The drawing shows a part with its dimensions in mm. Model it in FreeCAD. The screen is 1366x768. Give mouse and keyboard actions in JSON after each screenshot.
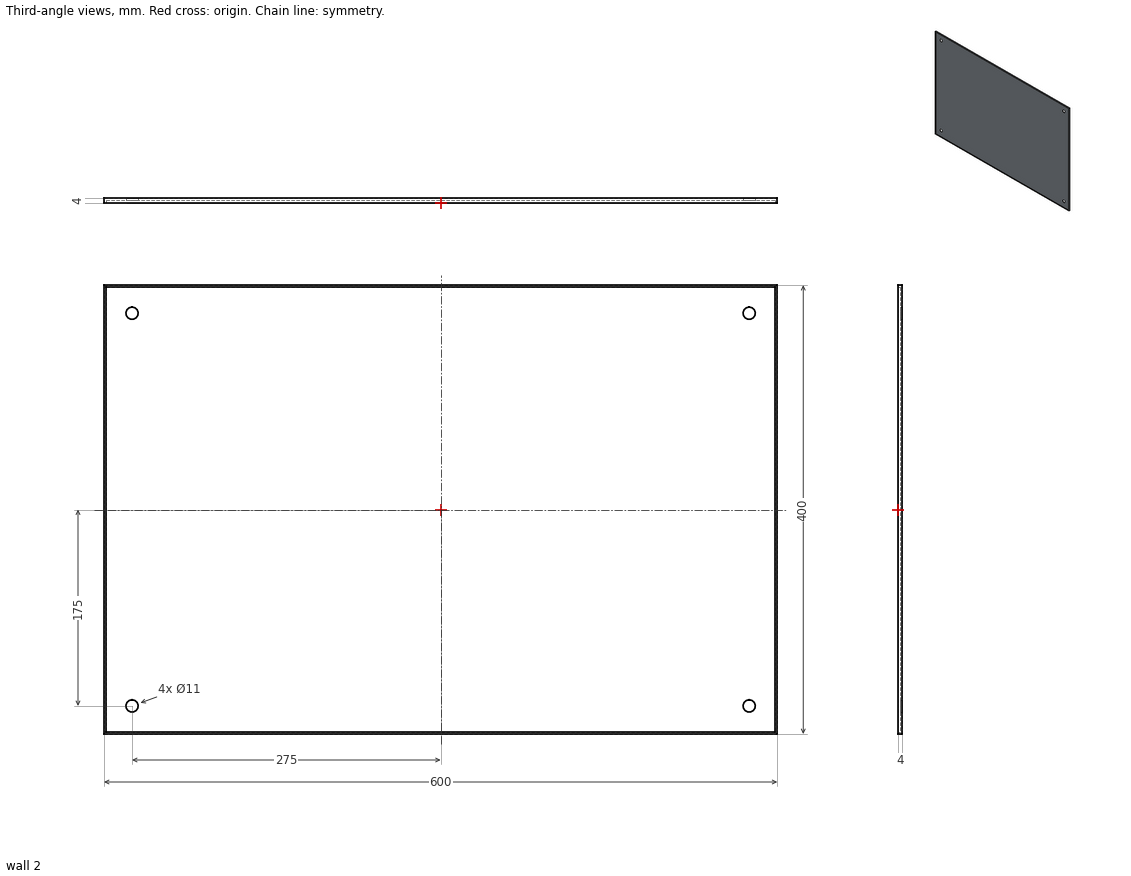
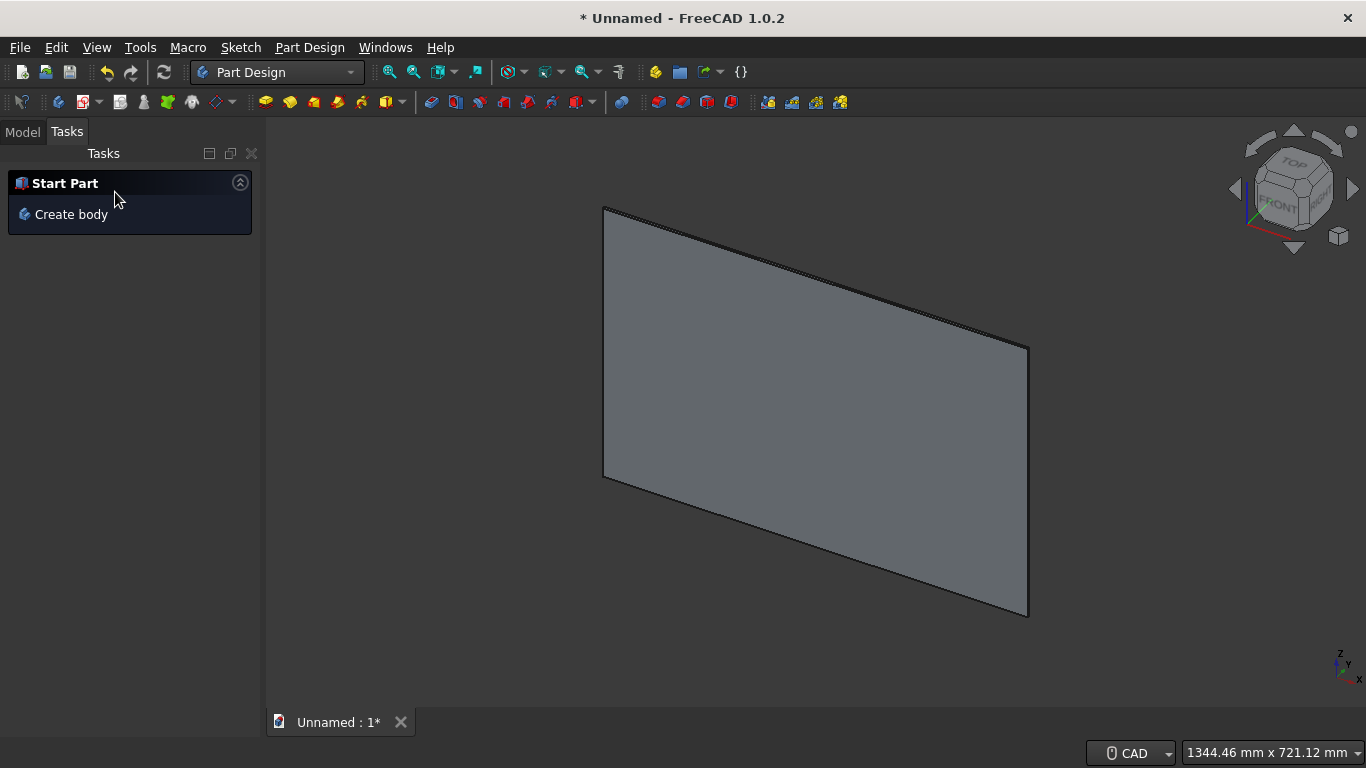
{"action": "left_click", "coordinate": [876, 432]}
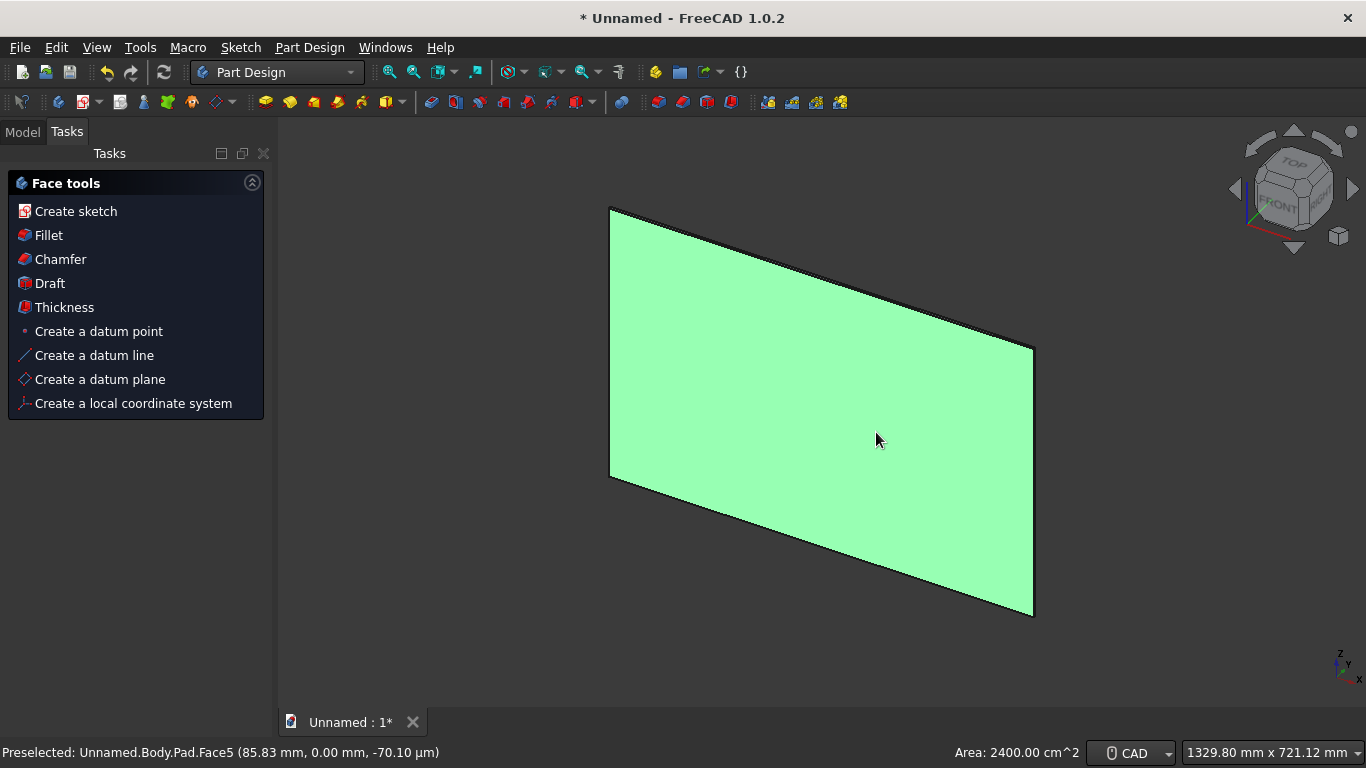
{"action": "left_click", "coordinate": [732, 102]}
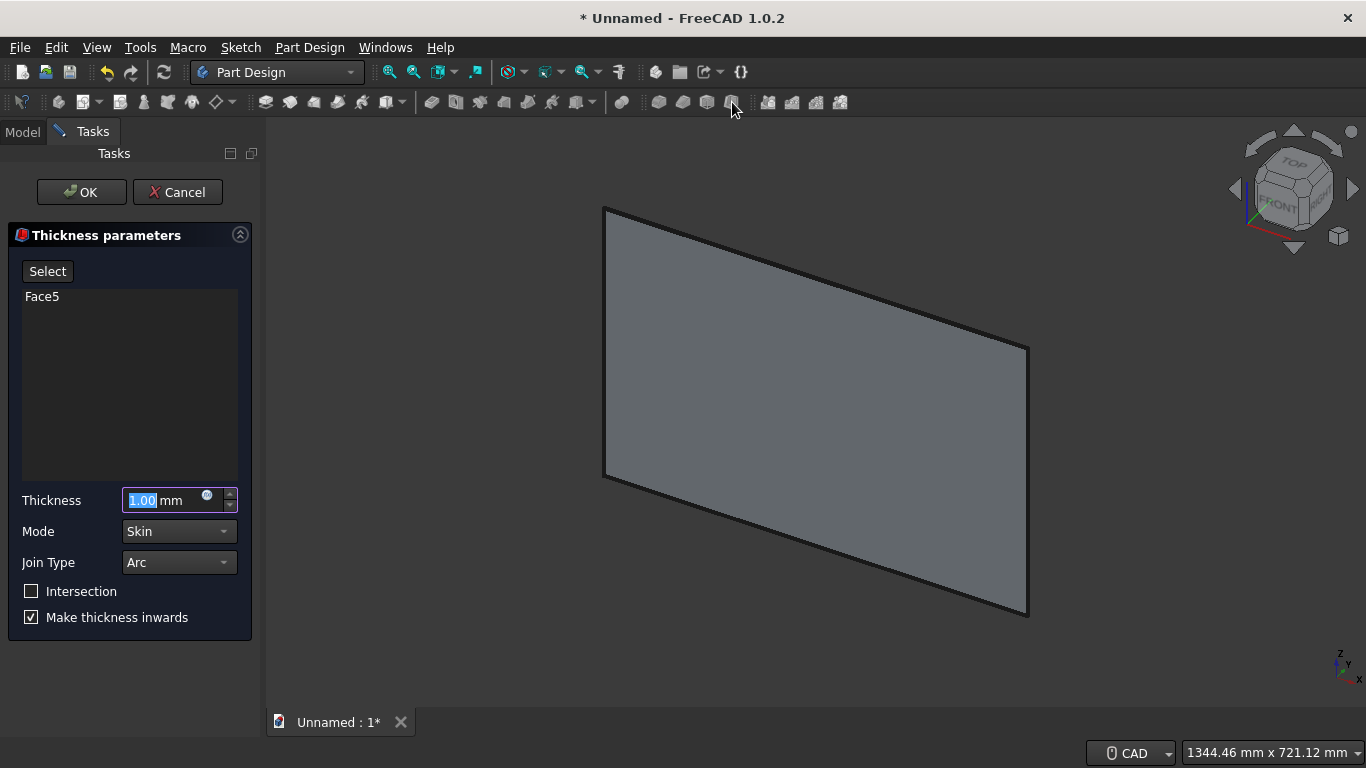
{"action": "type", "text": "2"}
{"action": "key", "text": "Tab"}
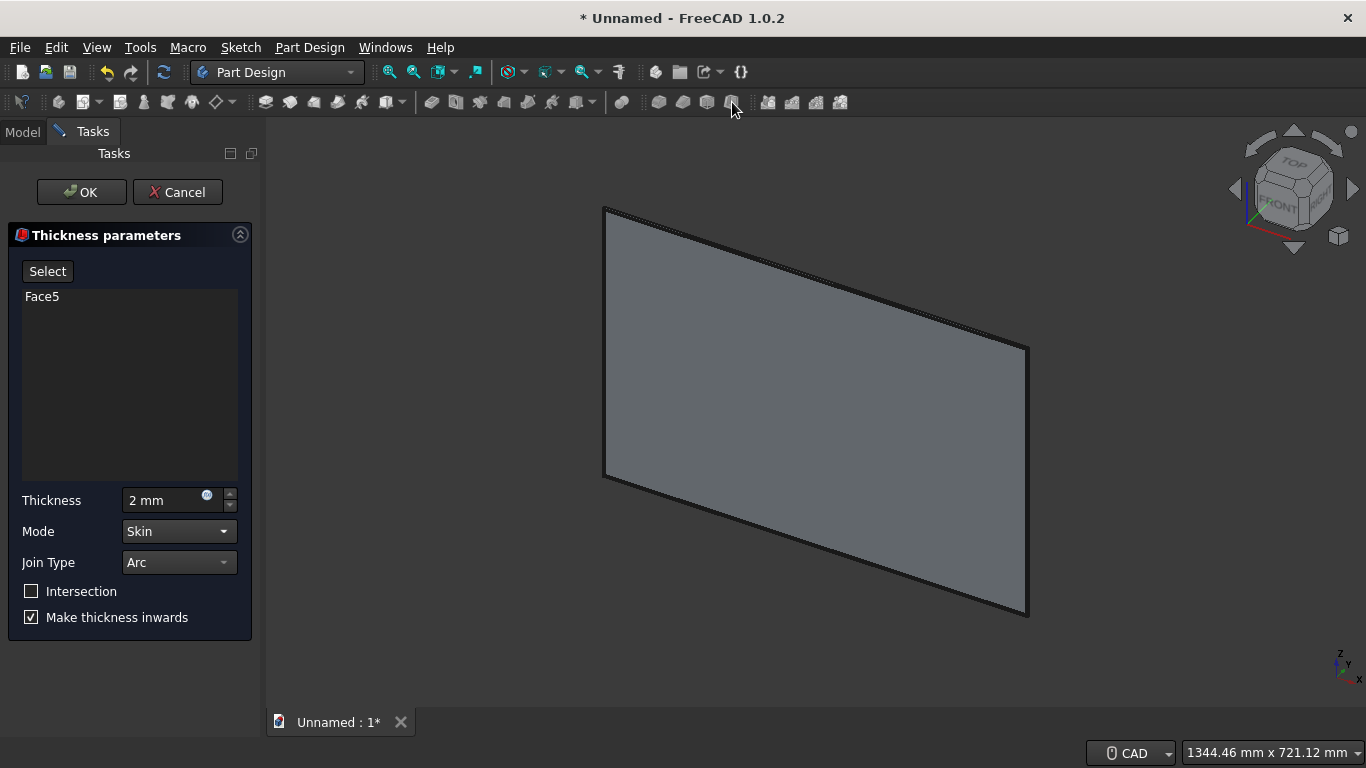
{"action": "left_click", "coordinate": [180, 562]}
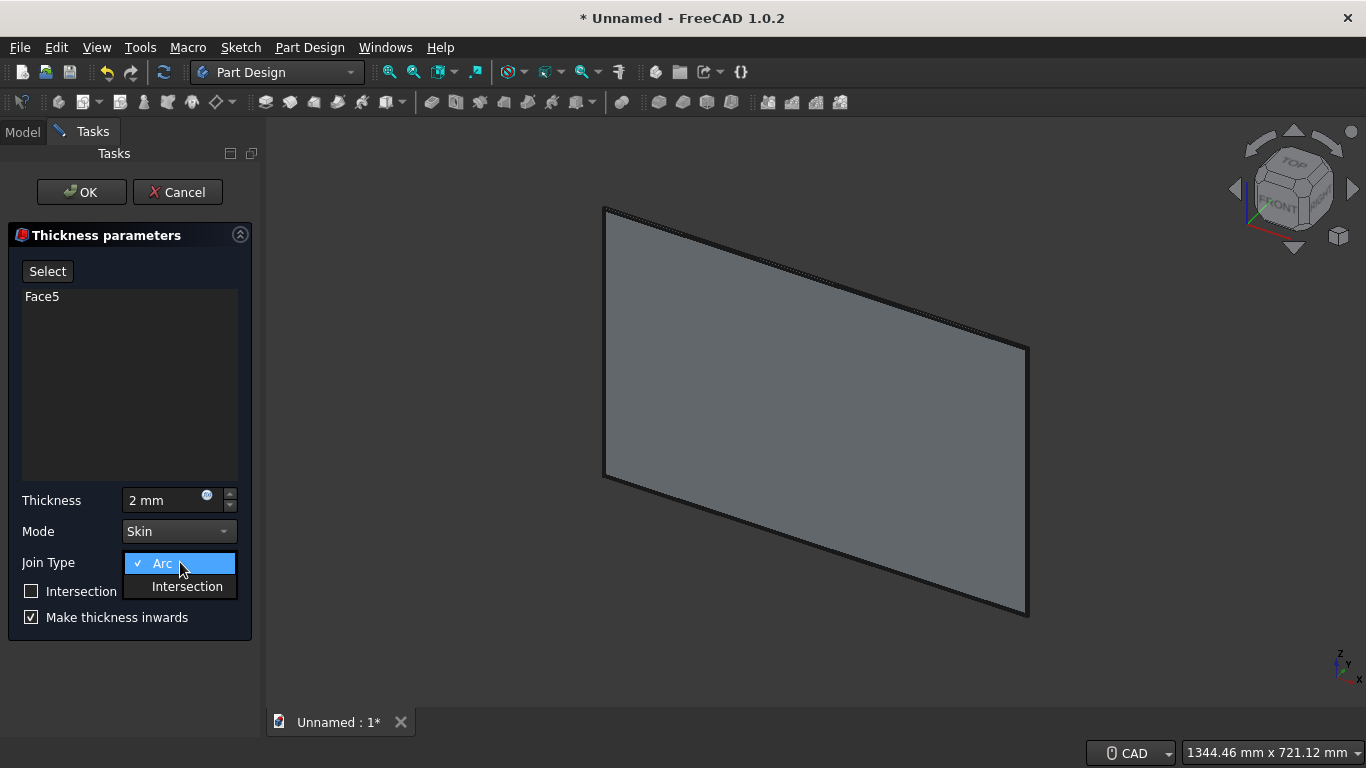
{"action": "left_click", "coordinate": [179, 586]}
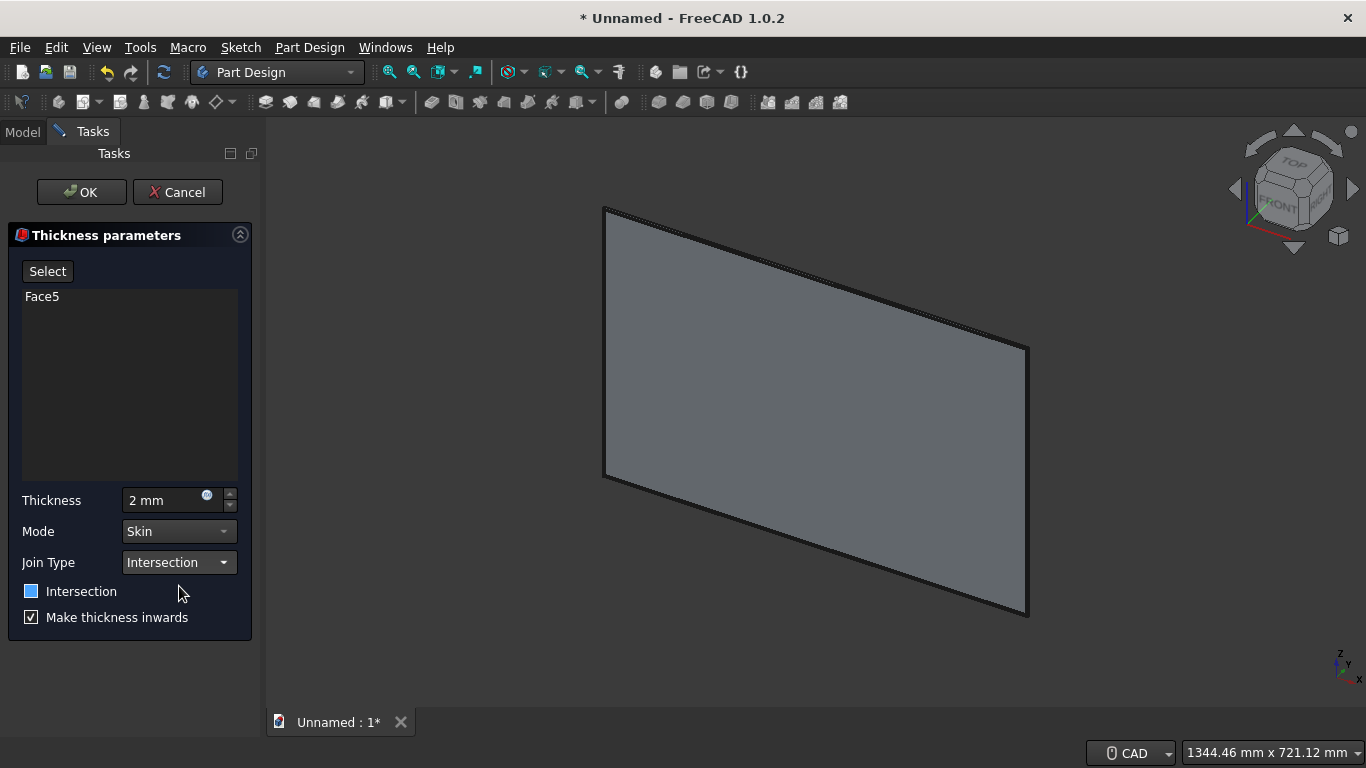
{"action": "left_click", "coordinate": [82, 192]}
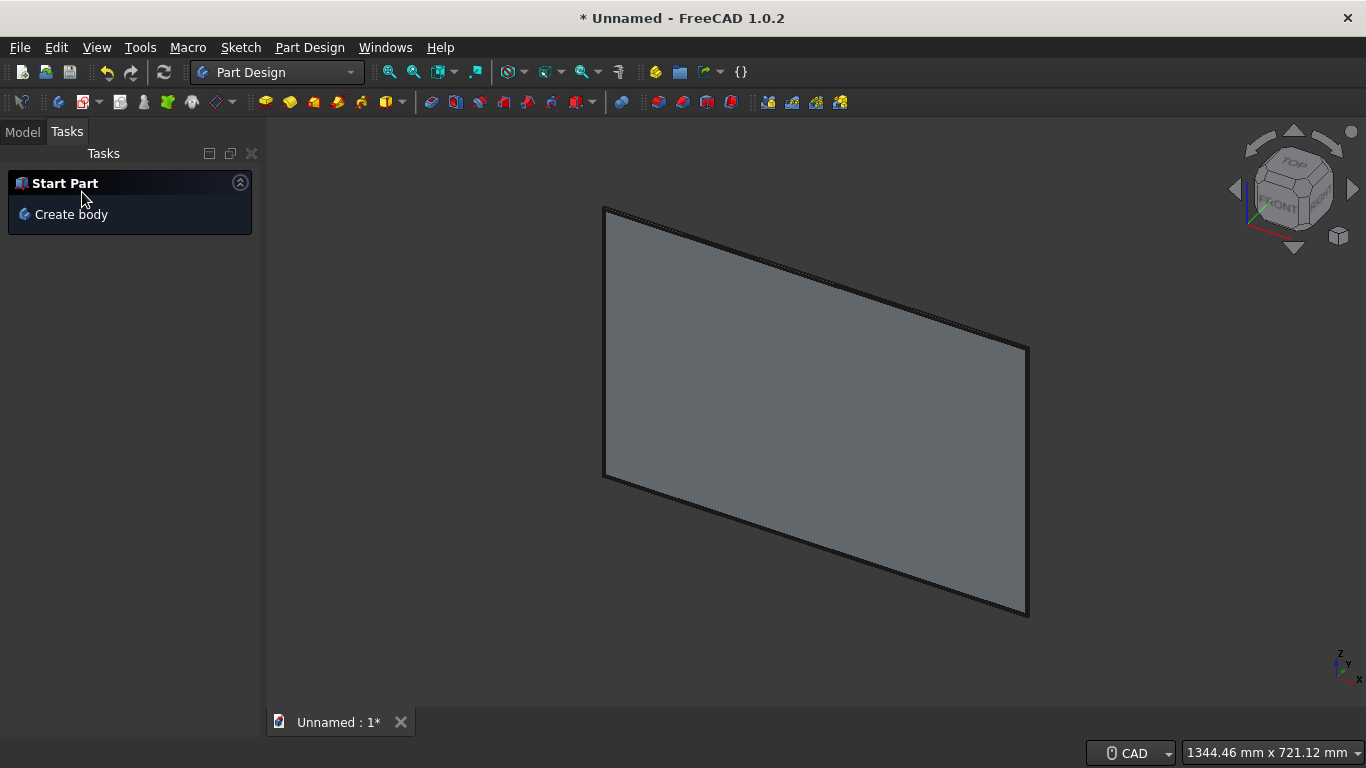
{"action": "key", "text": "4"}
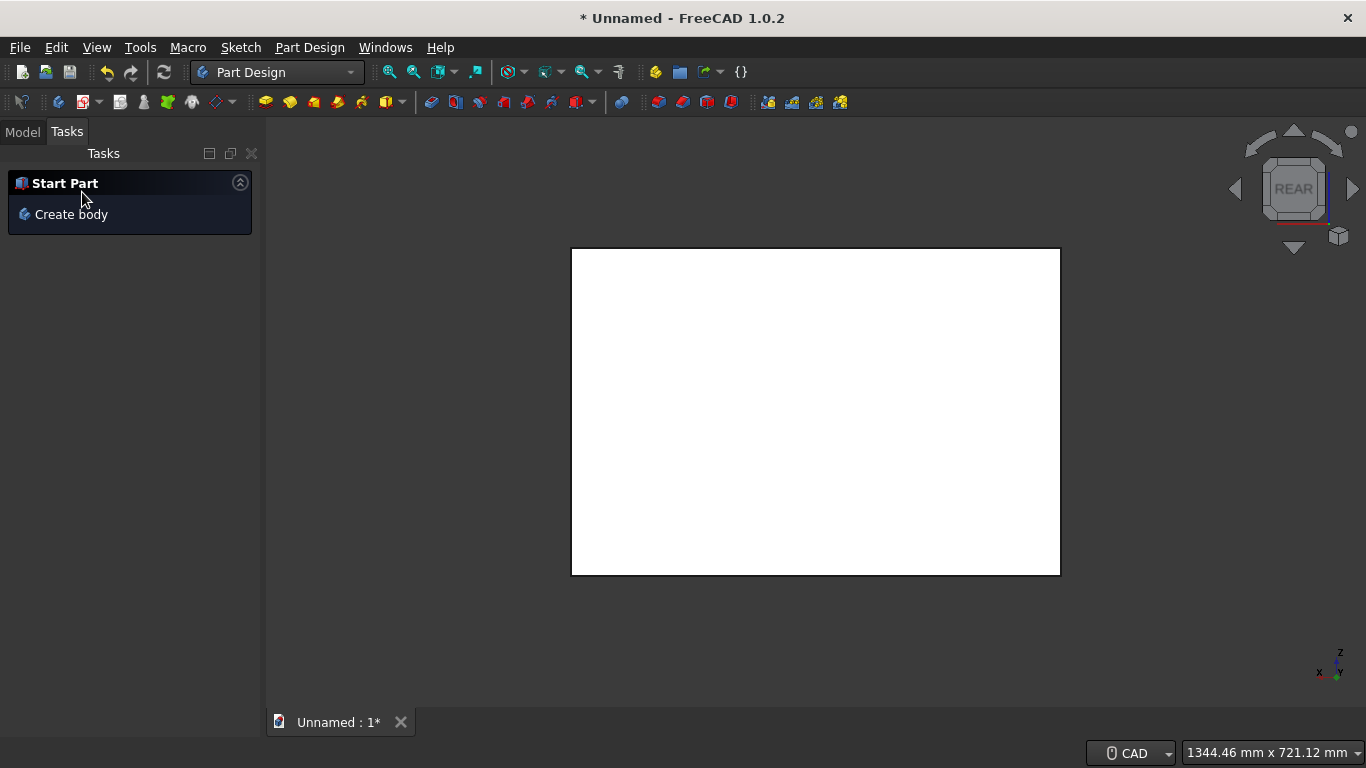
{"action": "left_click", "coordinate": [746, 411]}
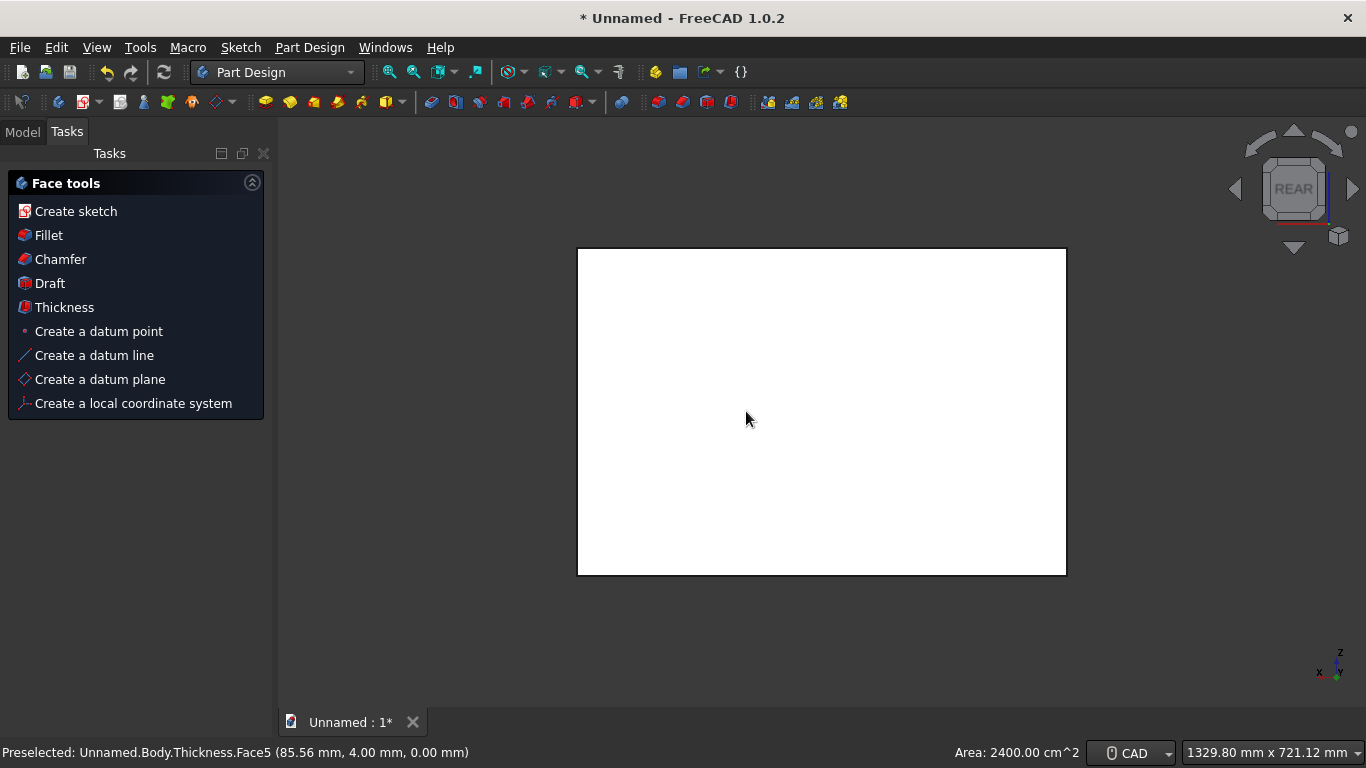
{"action": "left_click", "coordinate": [84, 102]}